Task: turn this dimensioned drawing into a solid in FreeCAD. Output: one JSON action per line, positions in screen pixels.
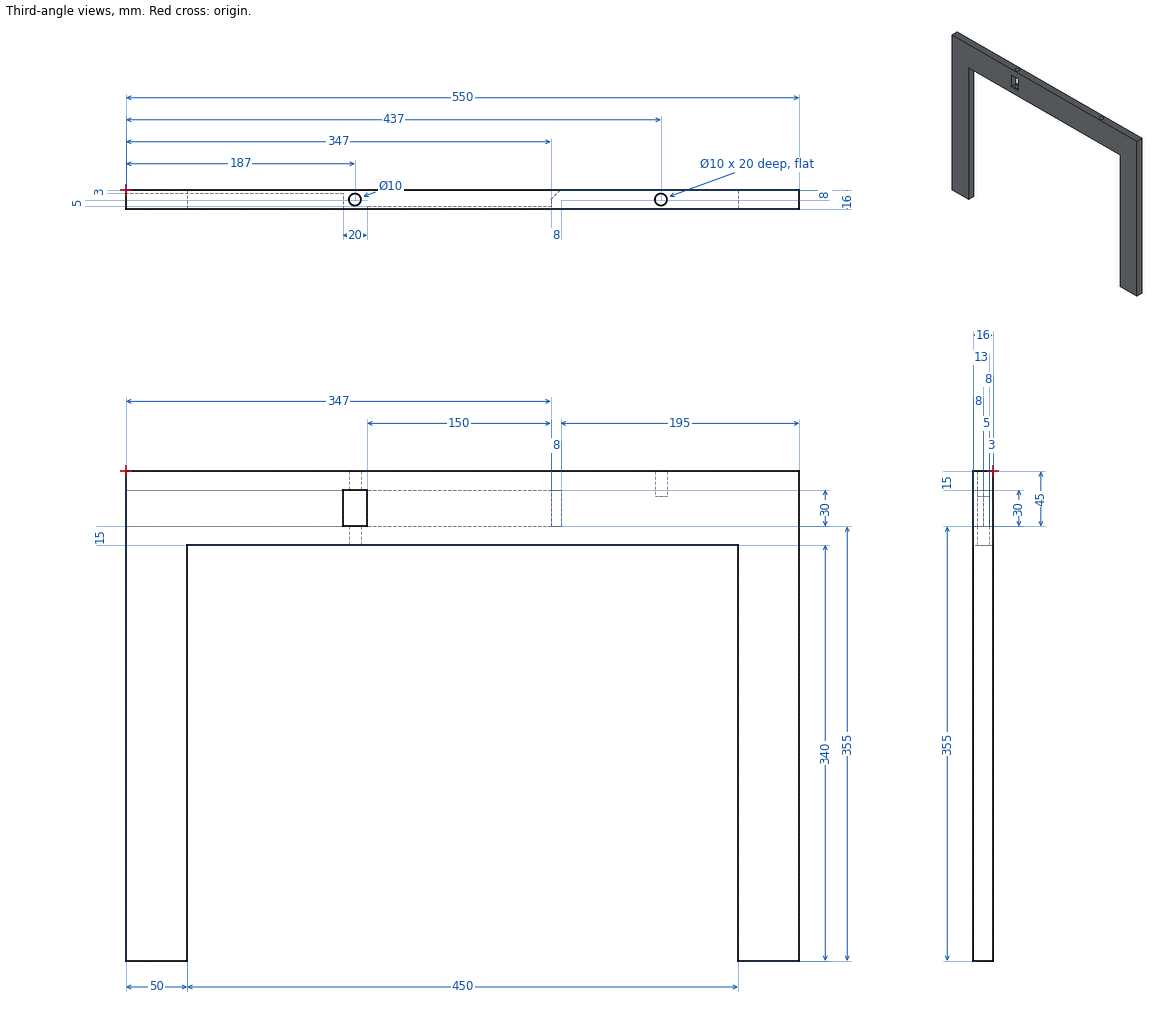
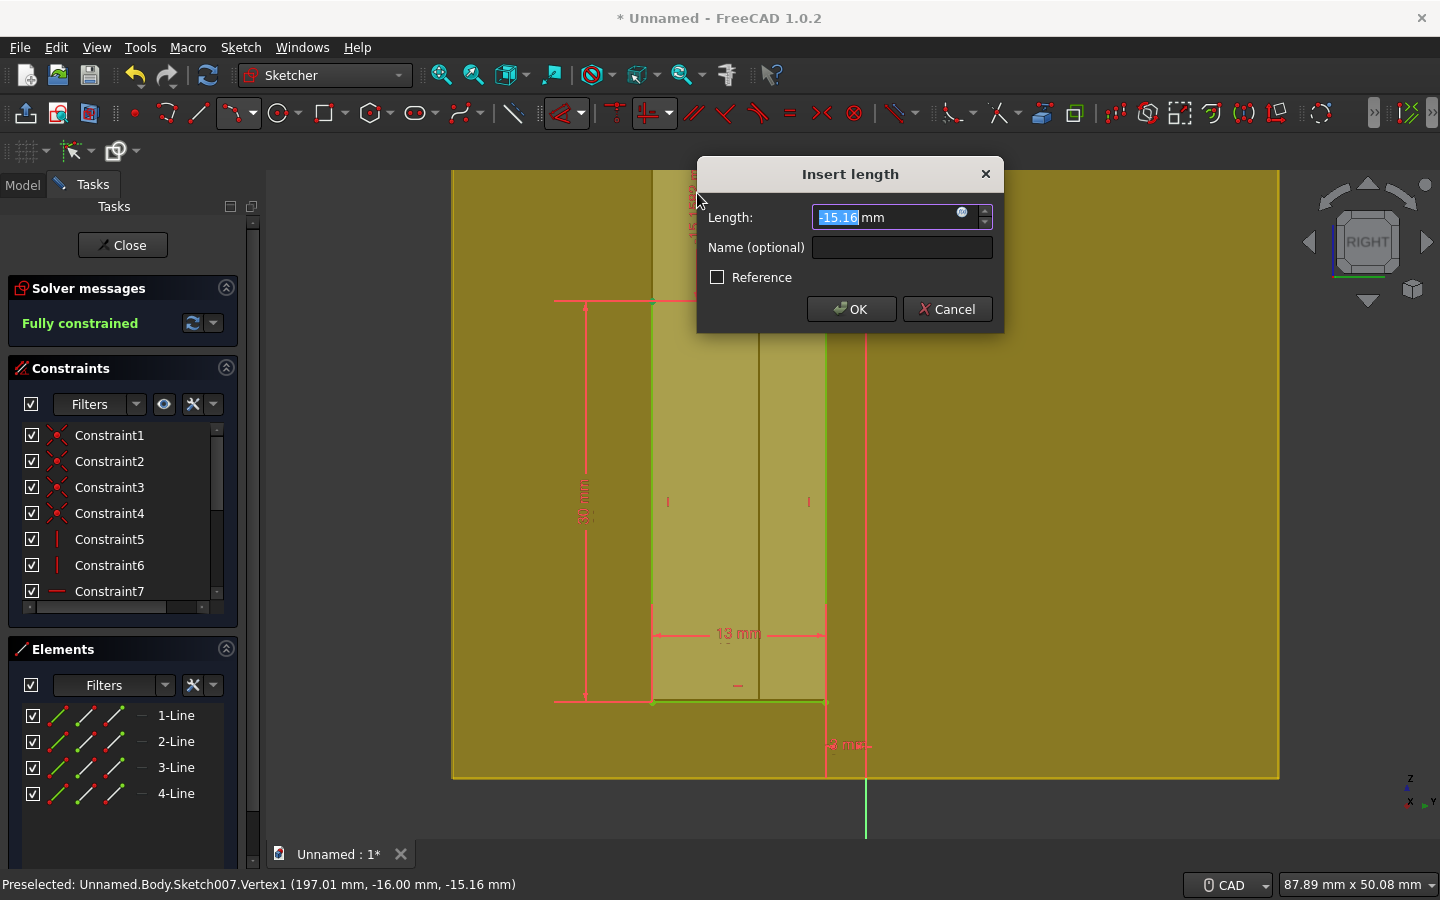
{"action": "type", "text": "-15"}
{"action": "key", "text": "Return"}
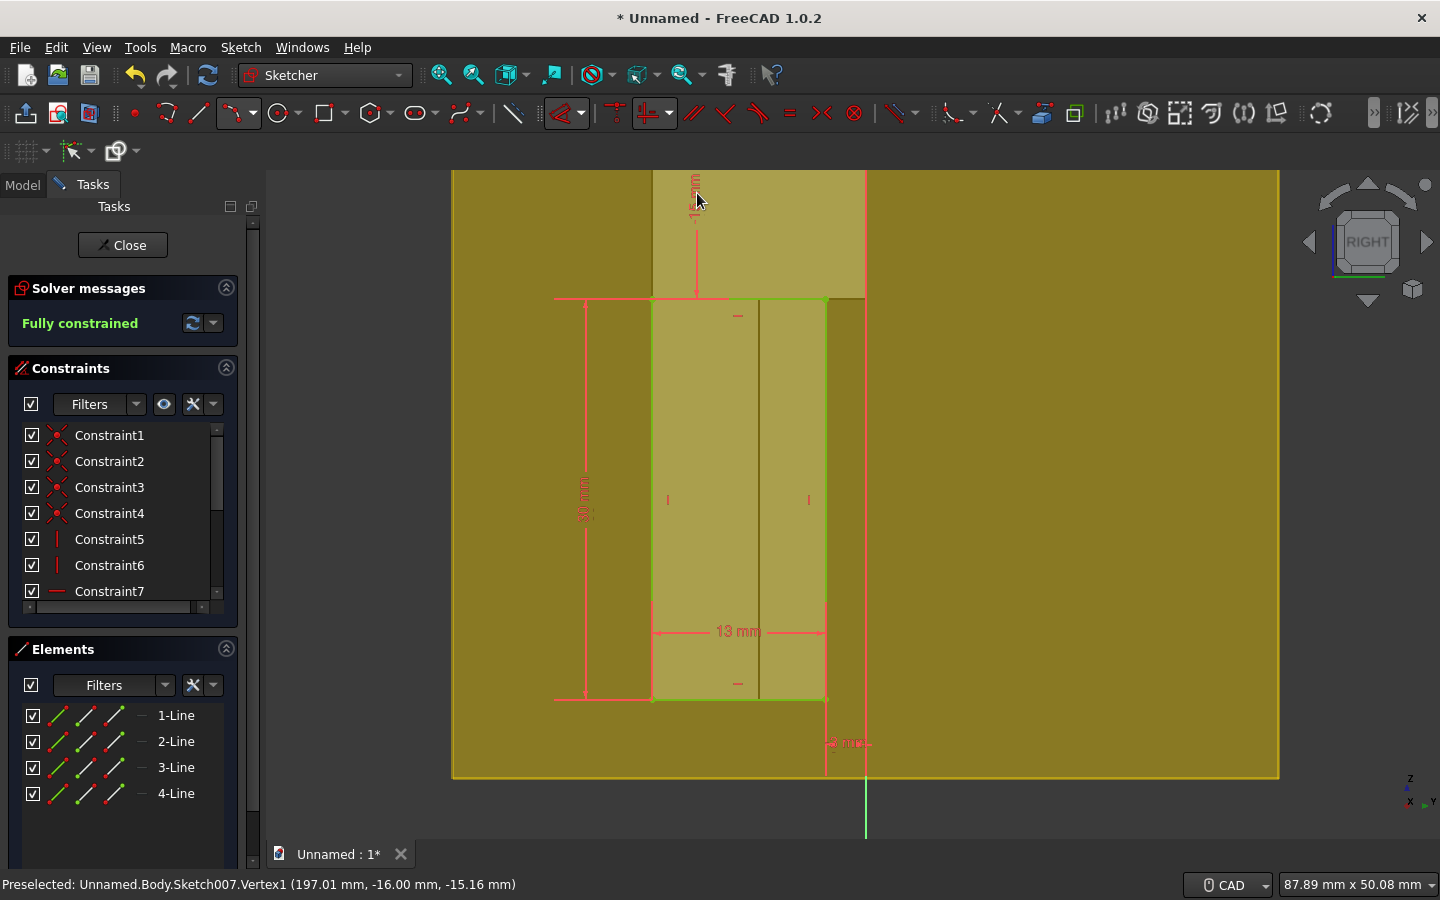
{"action": "left_click", "coordinate": [123, 245]}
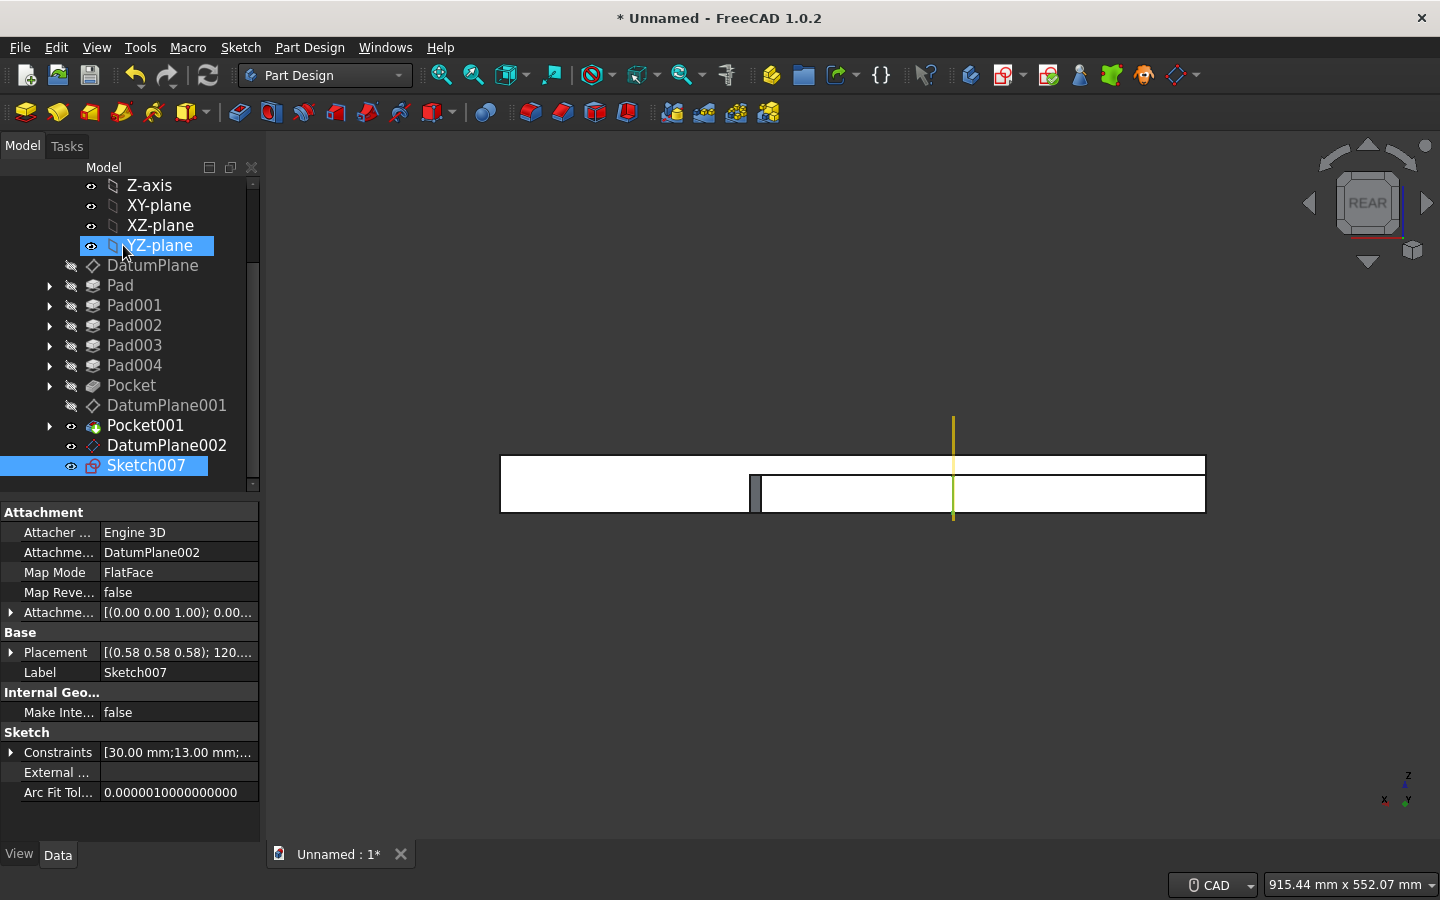
{"action": "left_click", "coordinate": [240, 112]}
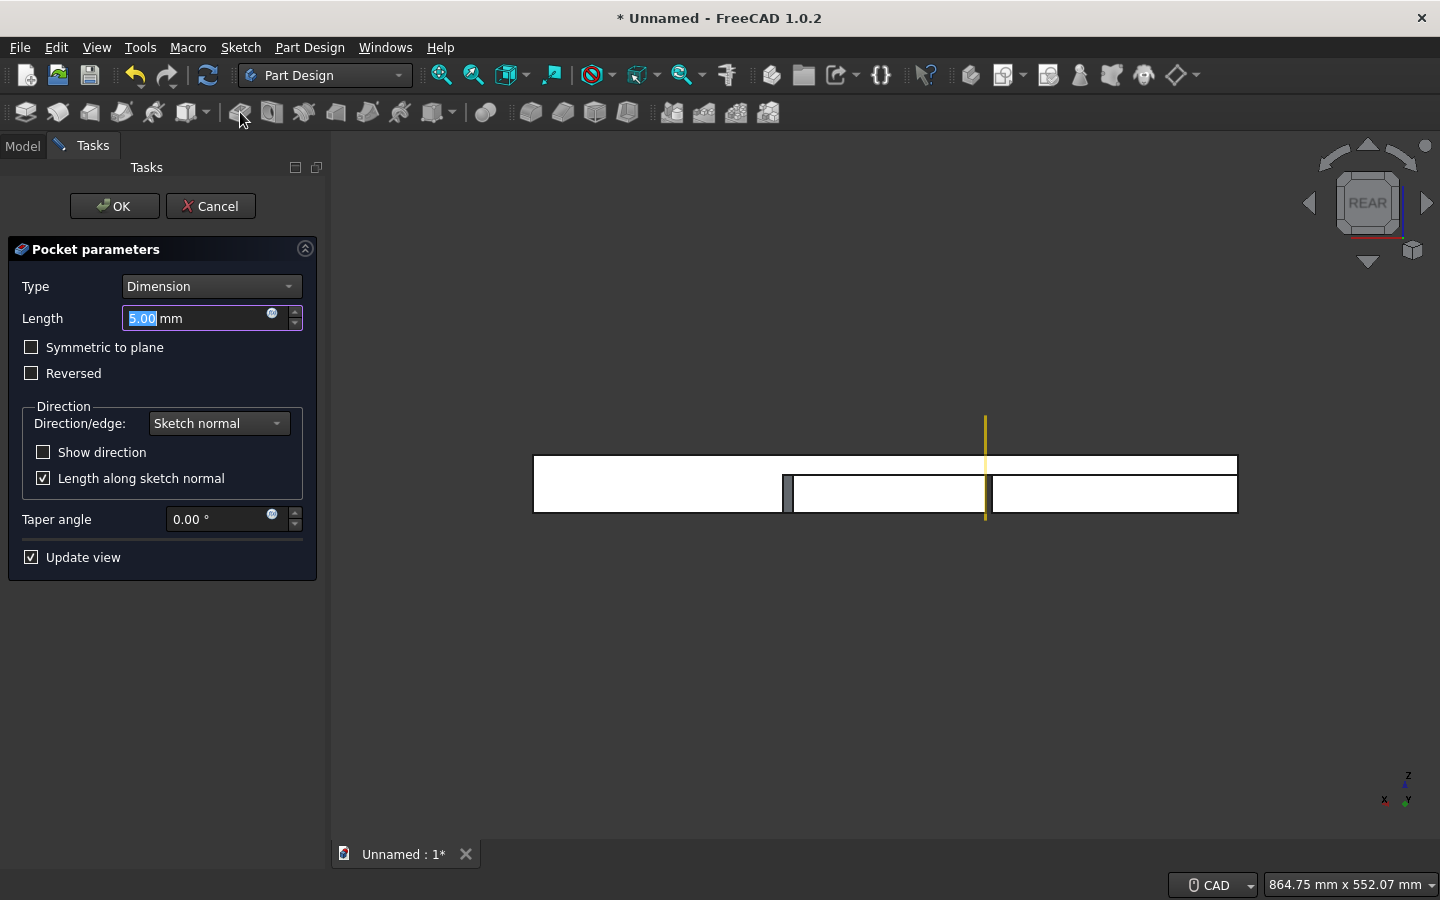
{"action": "type", "text": "20"}
{"action": "key", "text": "Tab"}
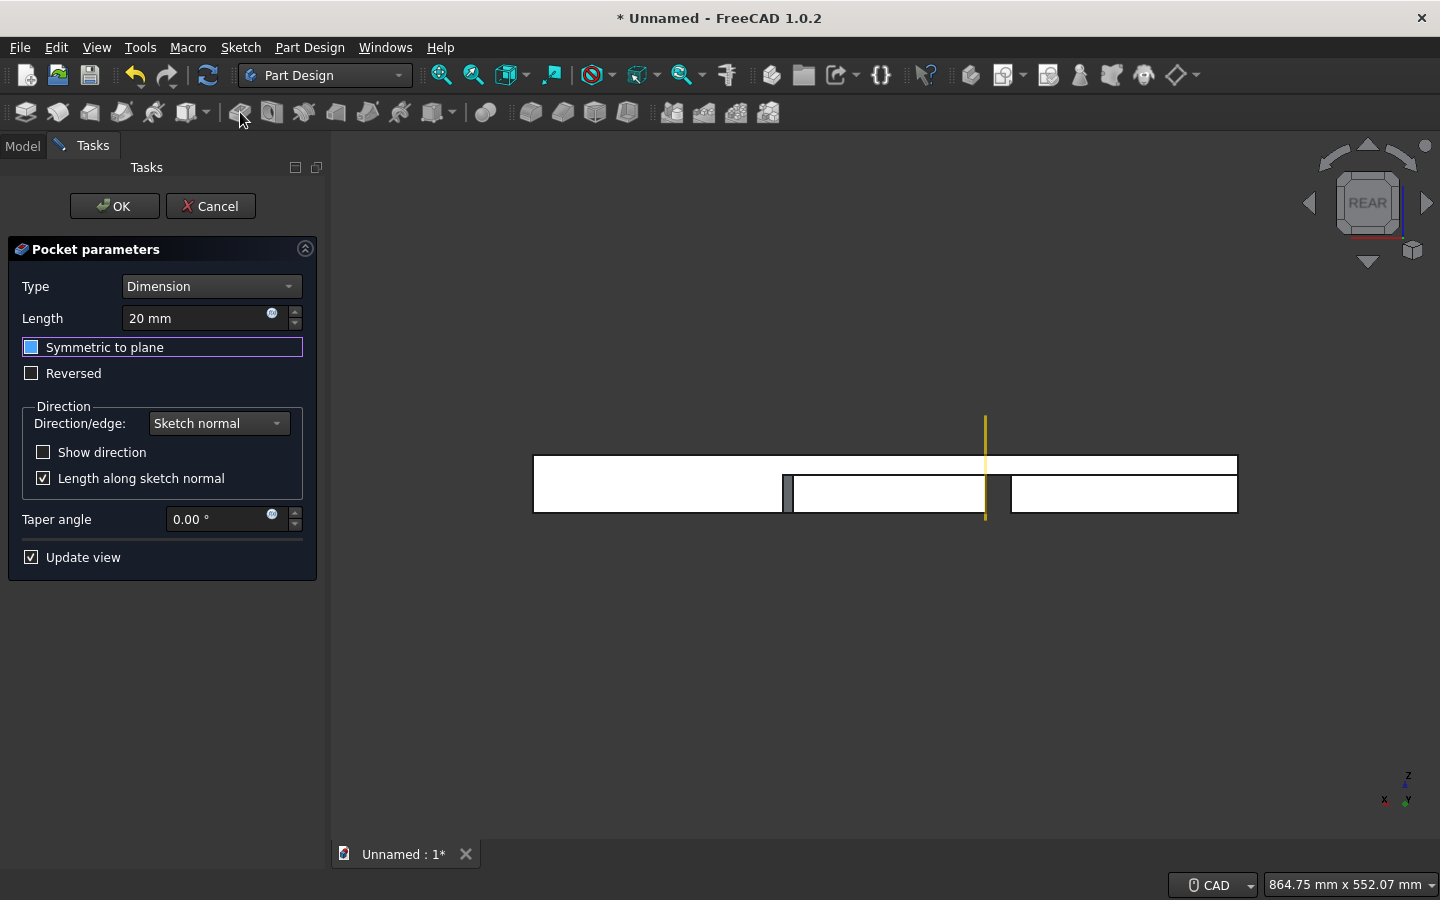
{"action": "left_click", "coordinate": [115, 206]}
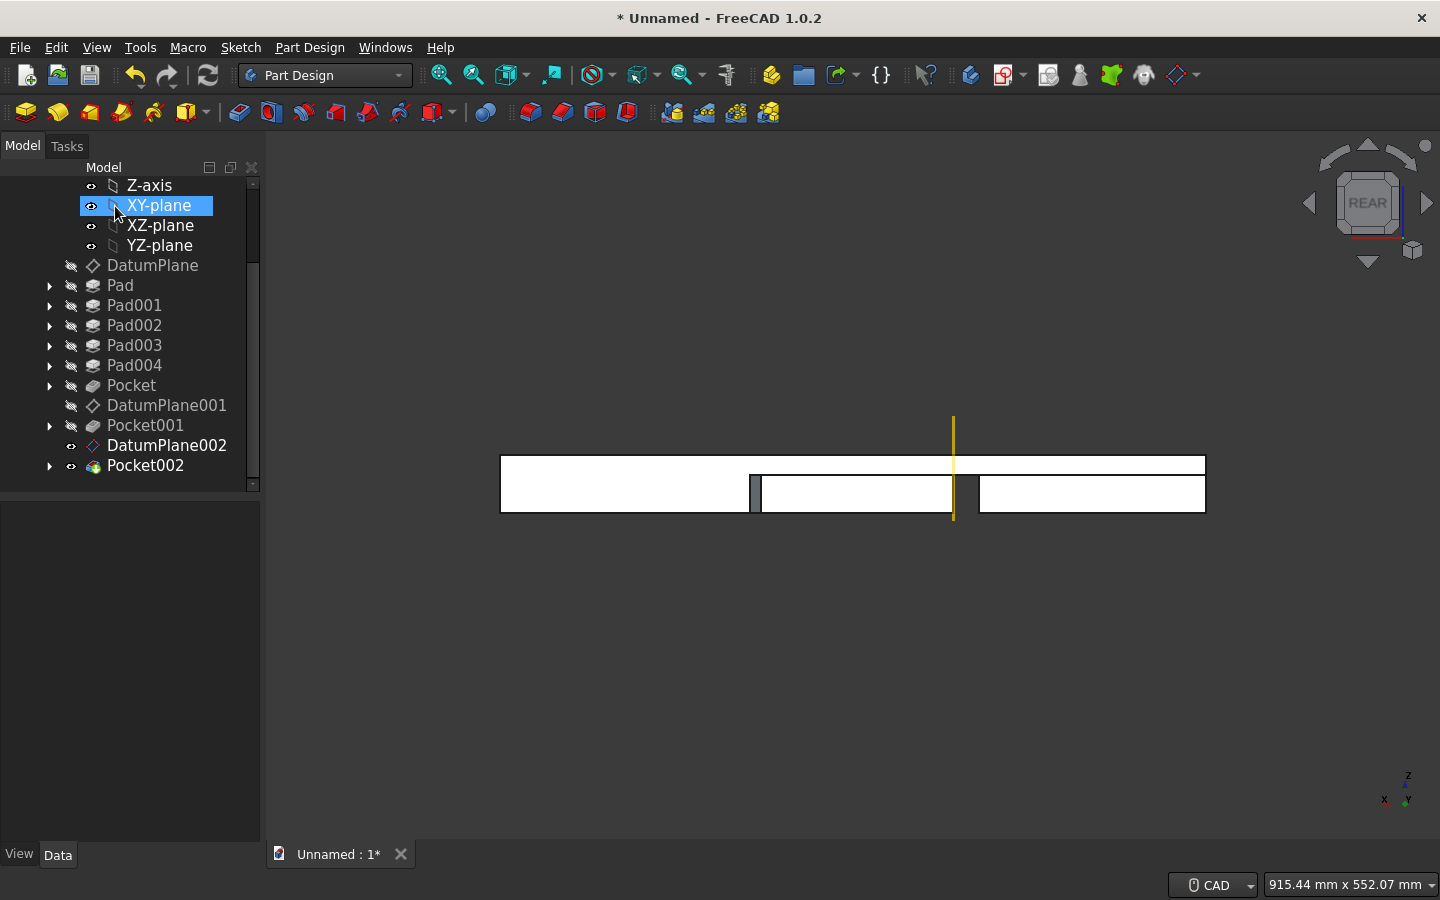
{"action": "left_click", "coordinate": [116, 446]}
{"action": "key", "text": "space"}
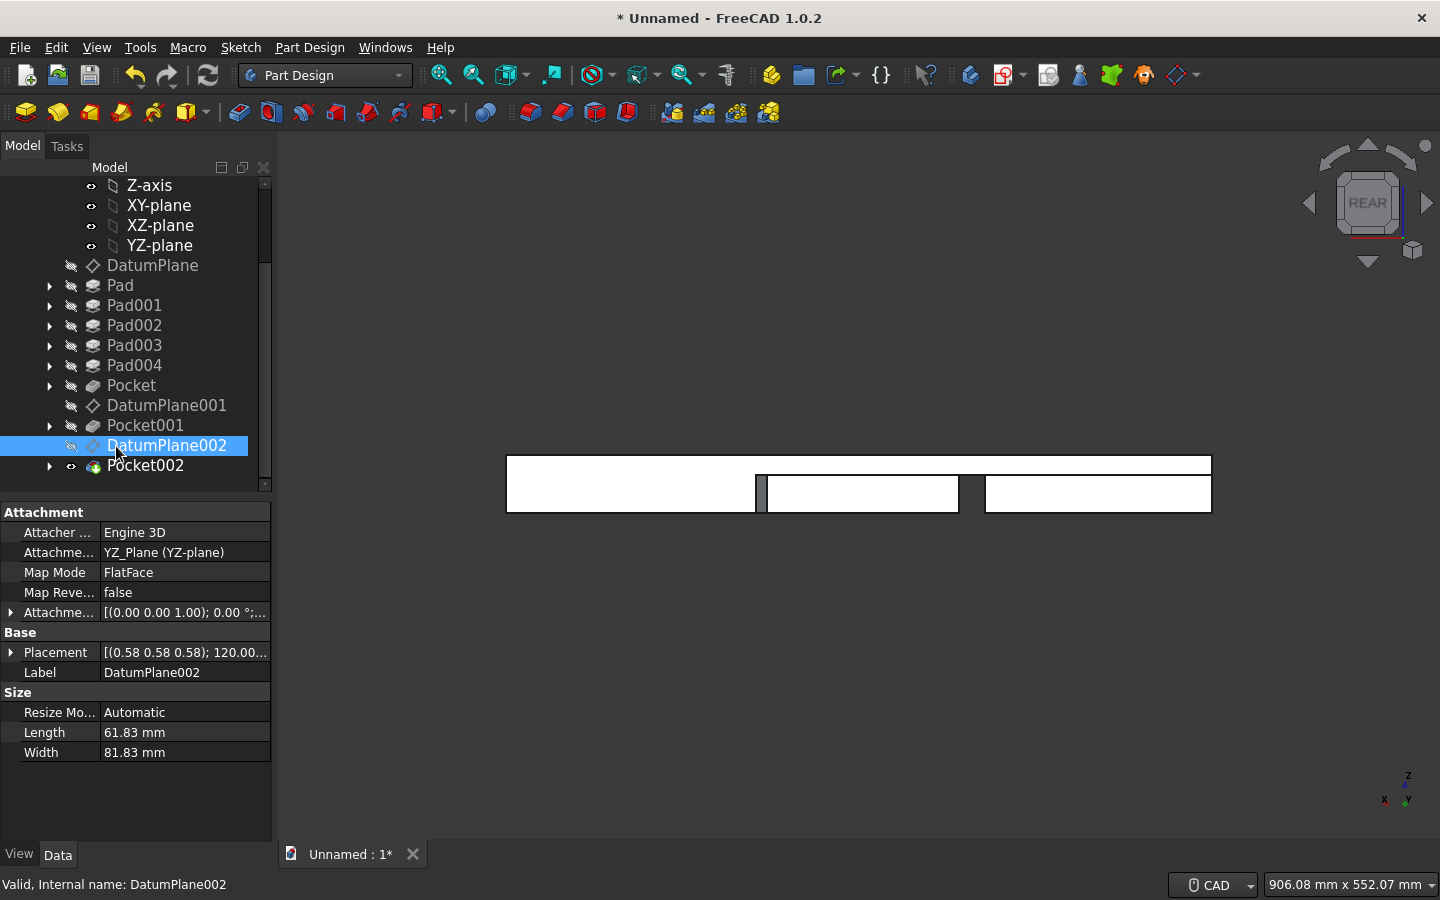
{"action": "left_click", "coordinate": [808, 493]}